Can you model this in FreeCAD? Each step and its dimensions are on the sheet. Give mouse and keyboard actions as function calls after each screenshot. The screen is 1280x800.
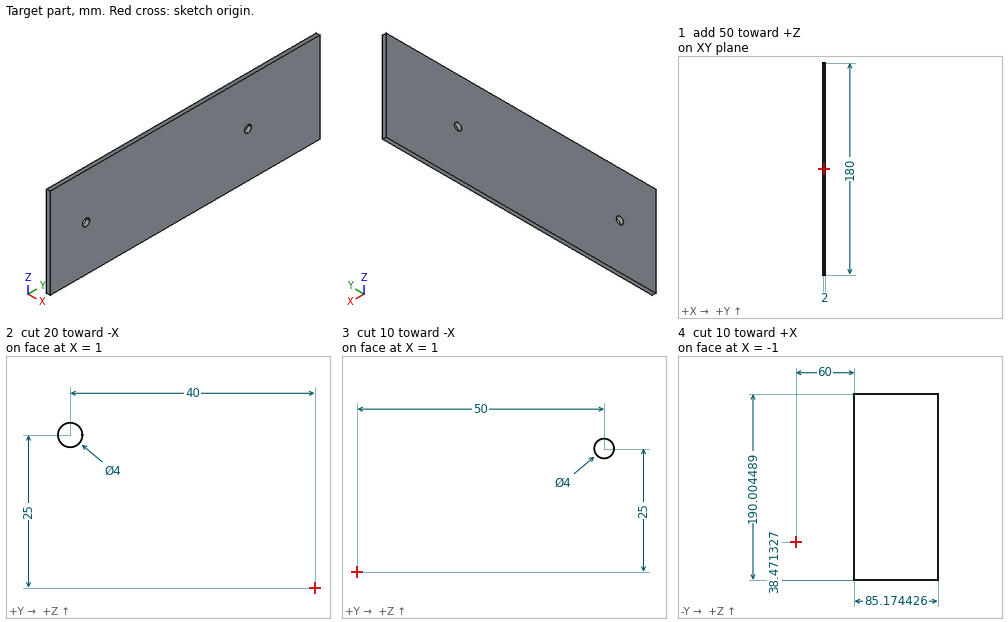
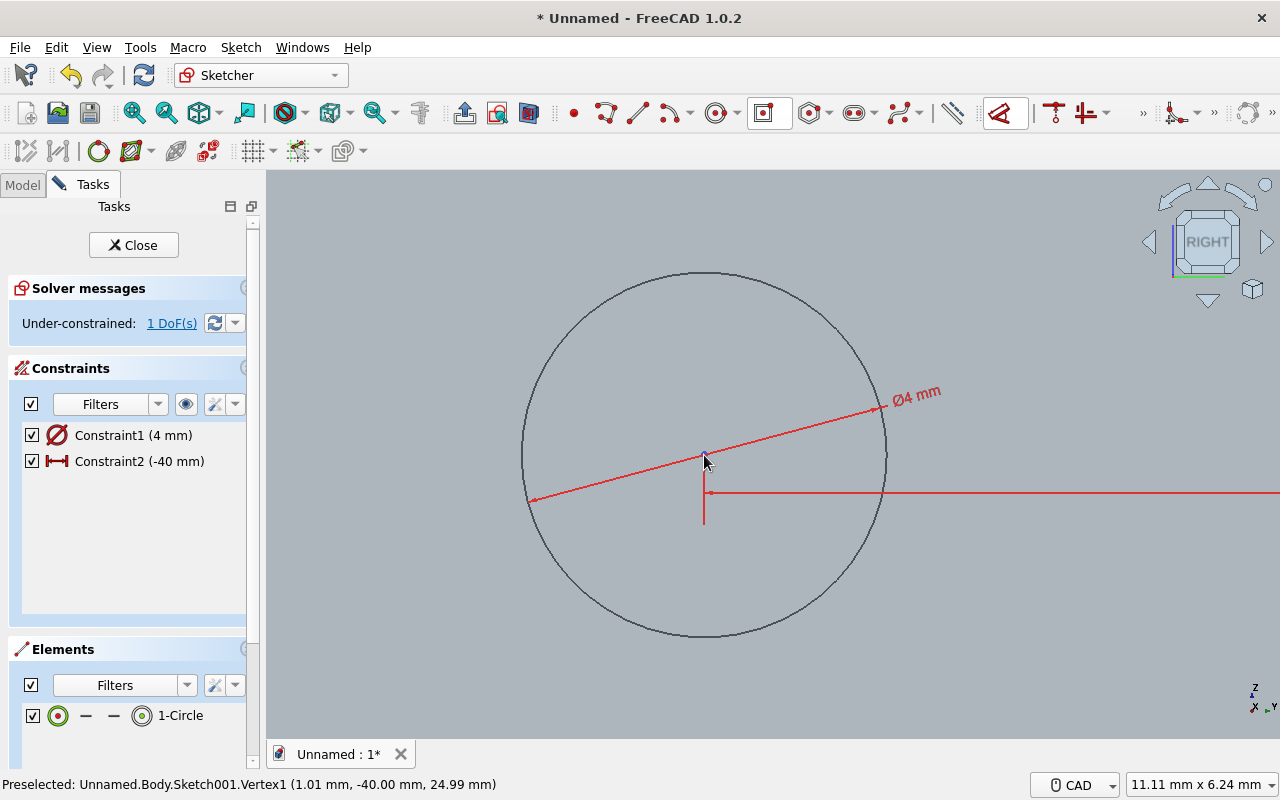
click(704, 455)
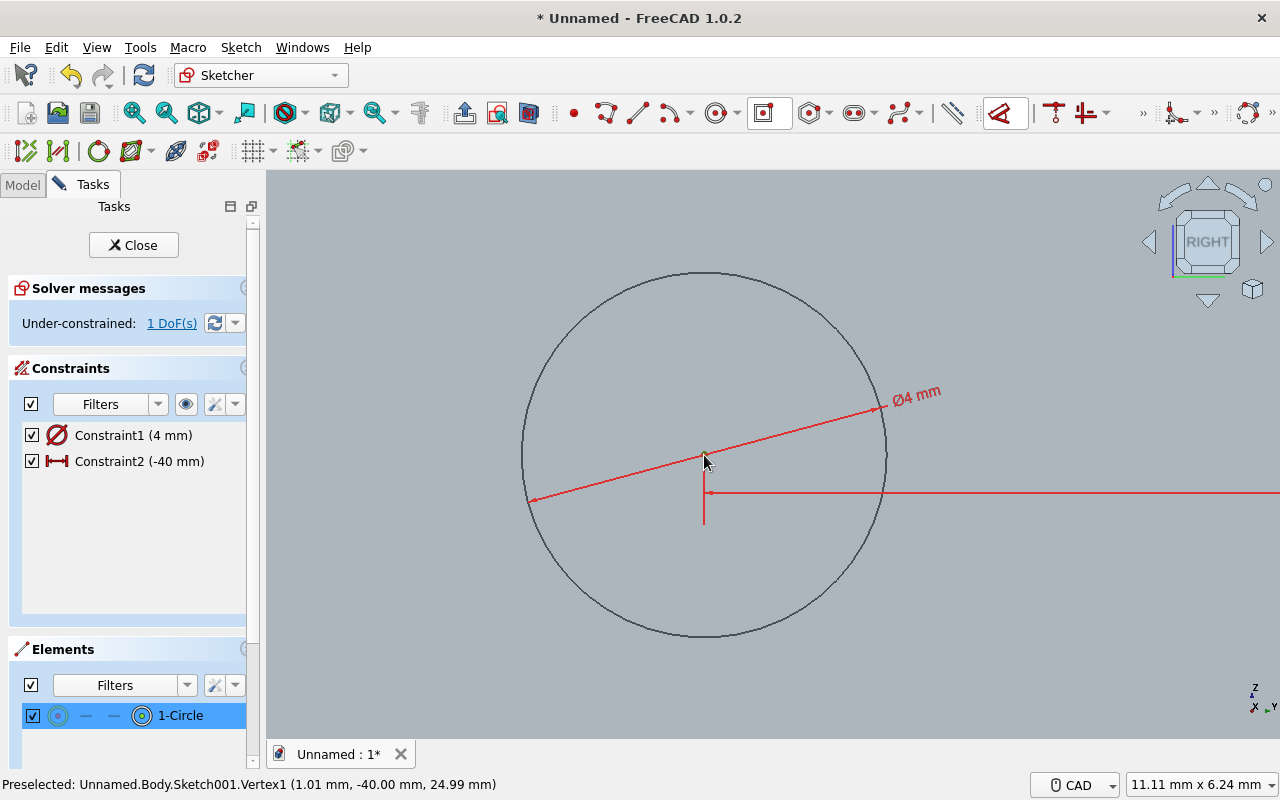
click(1022, 114)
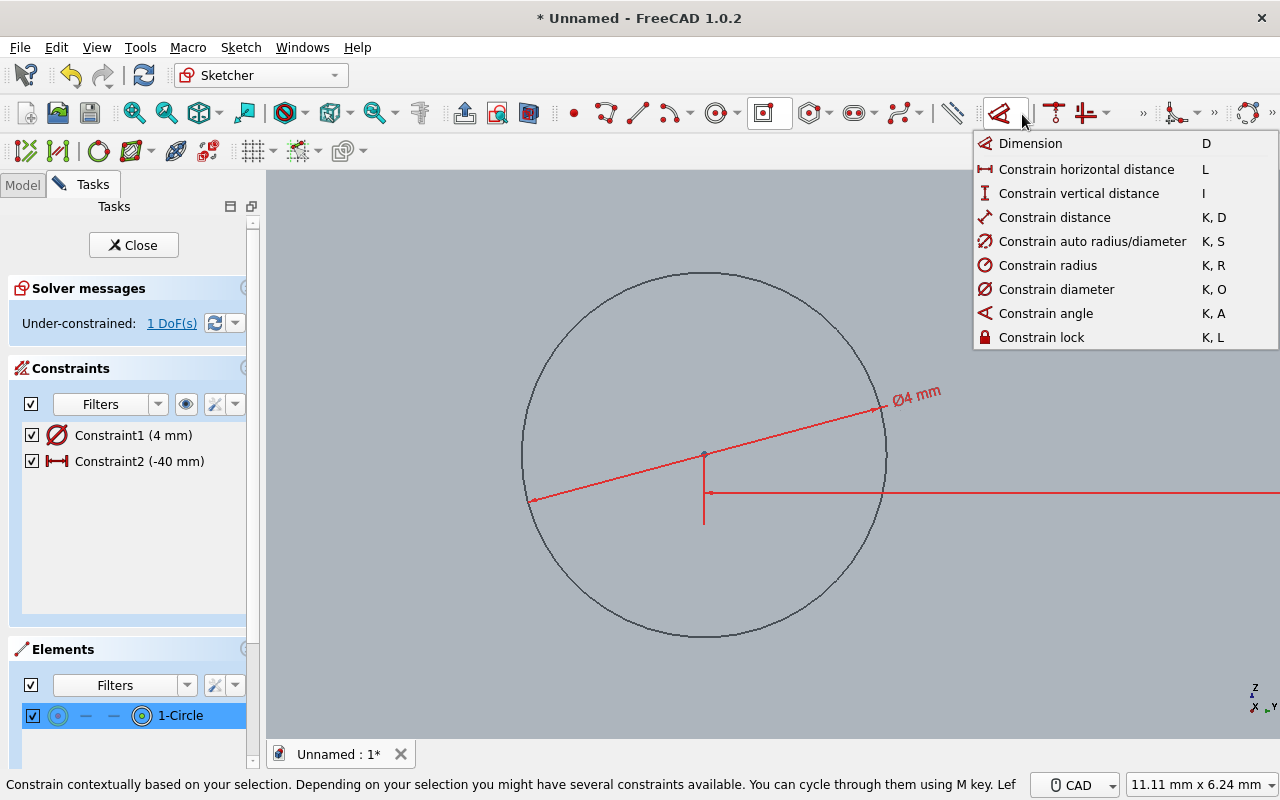
click(1126, 193)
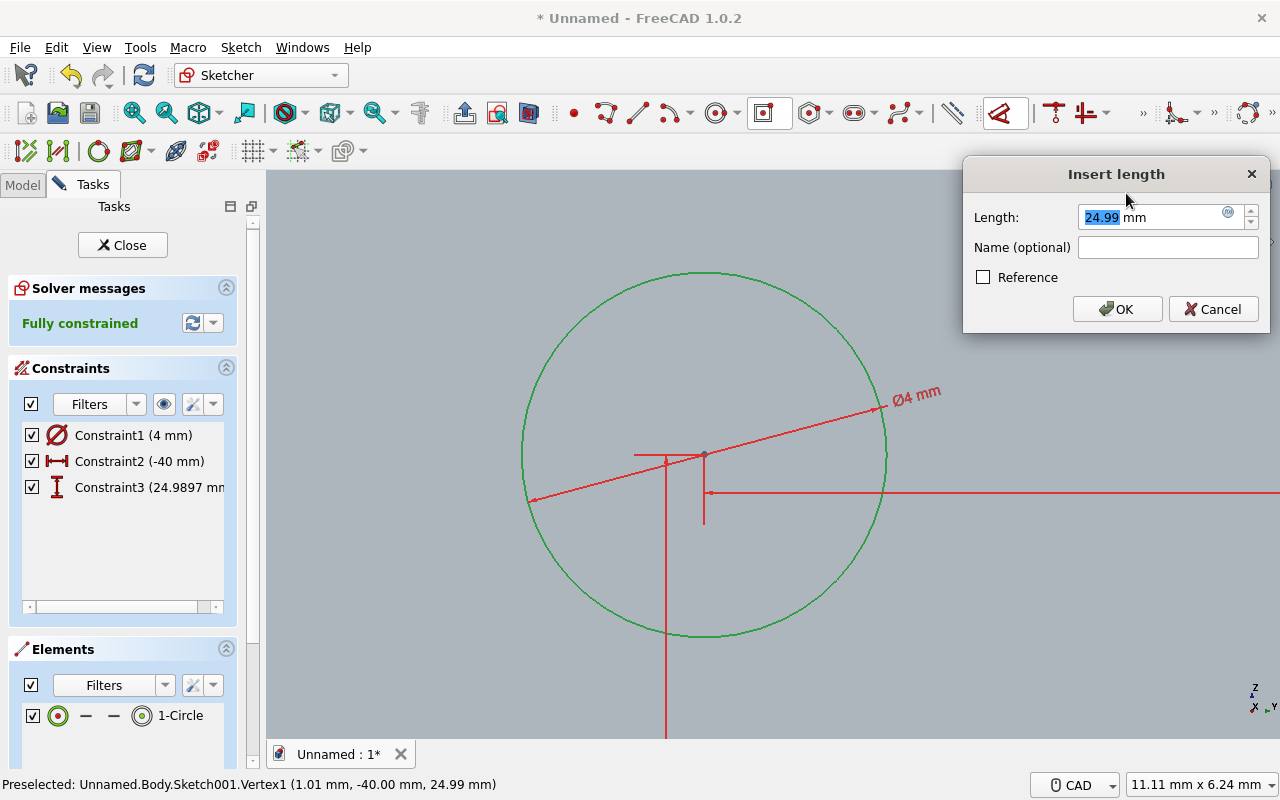
text(25)
key(Return)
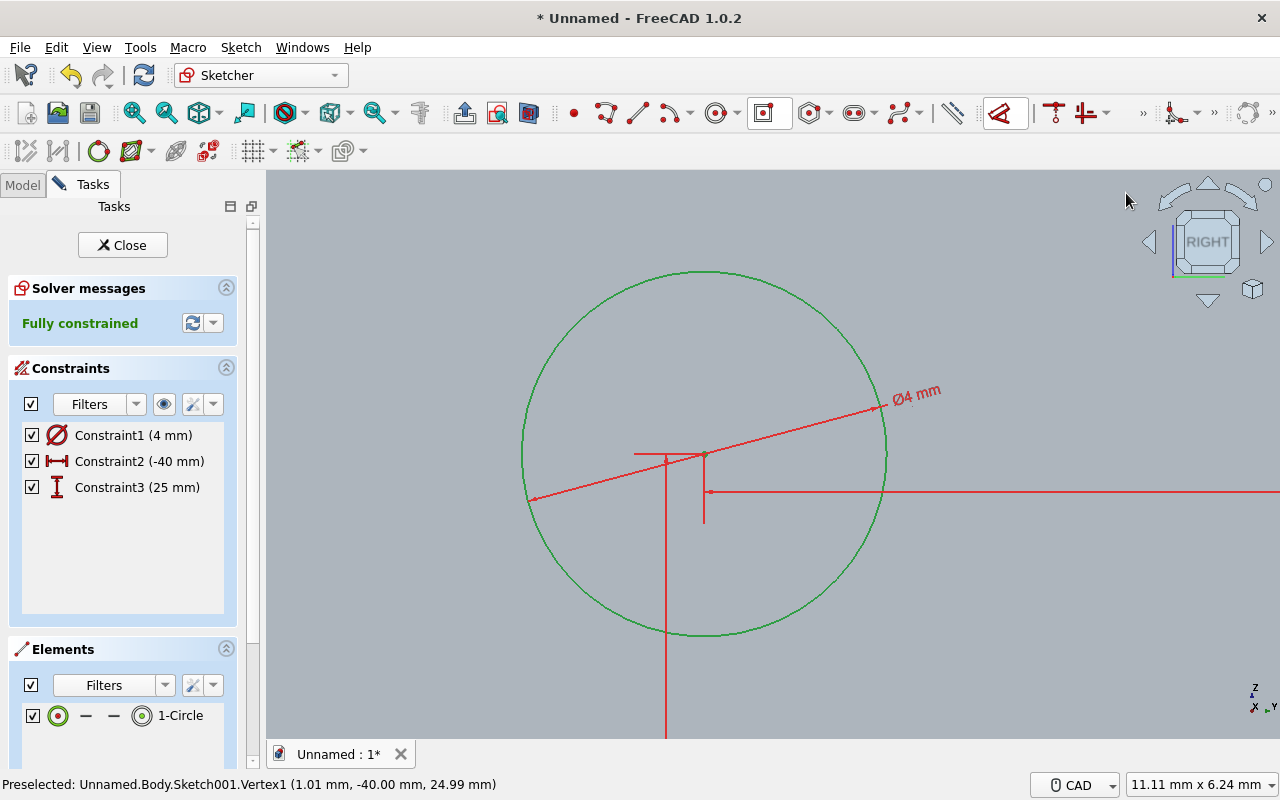
click(123, 245)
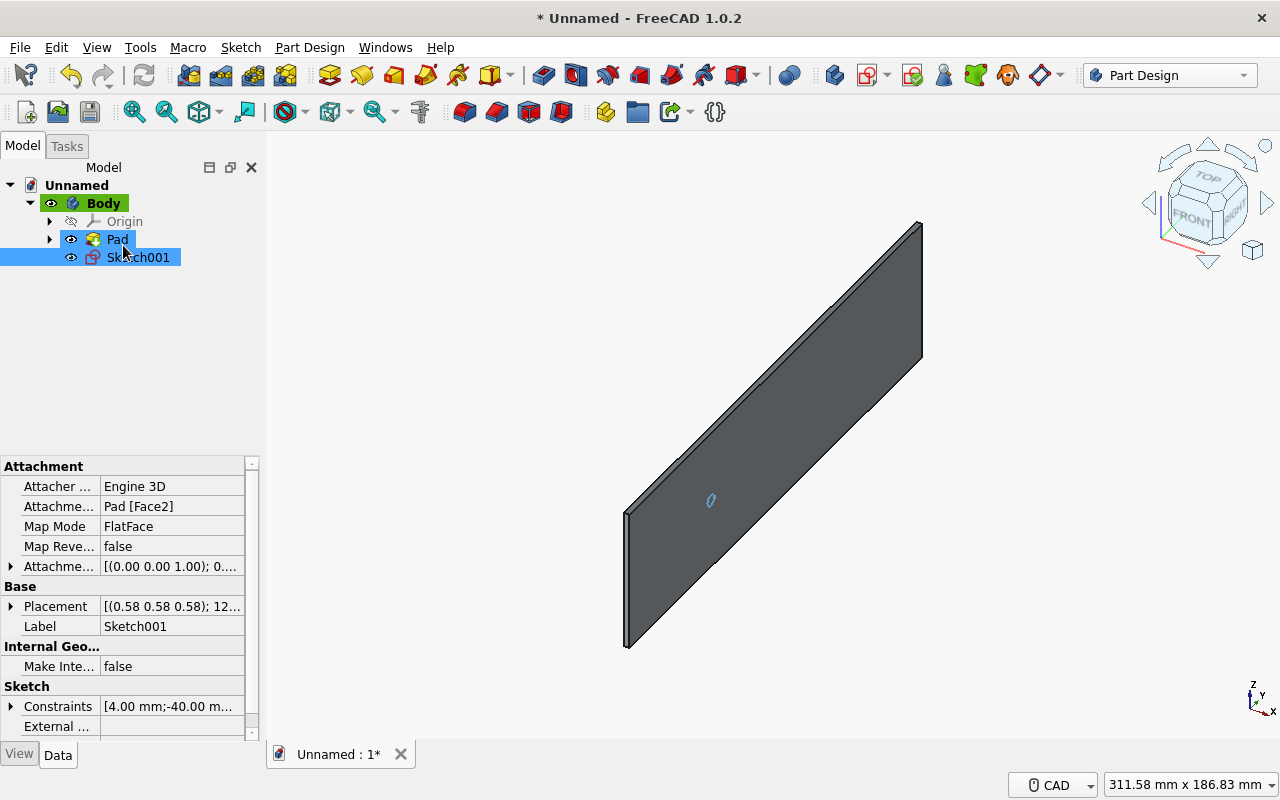
click(544, 76)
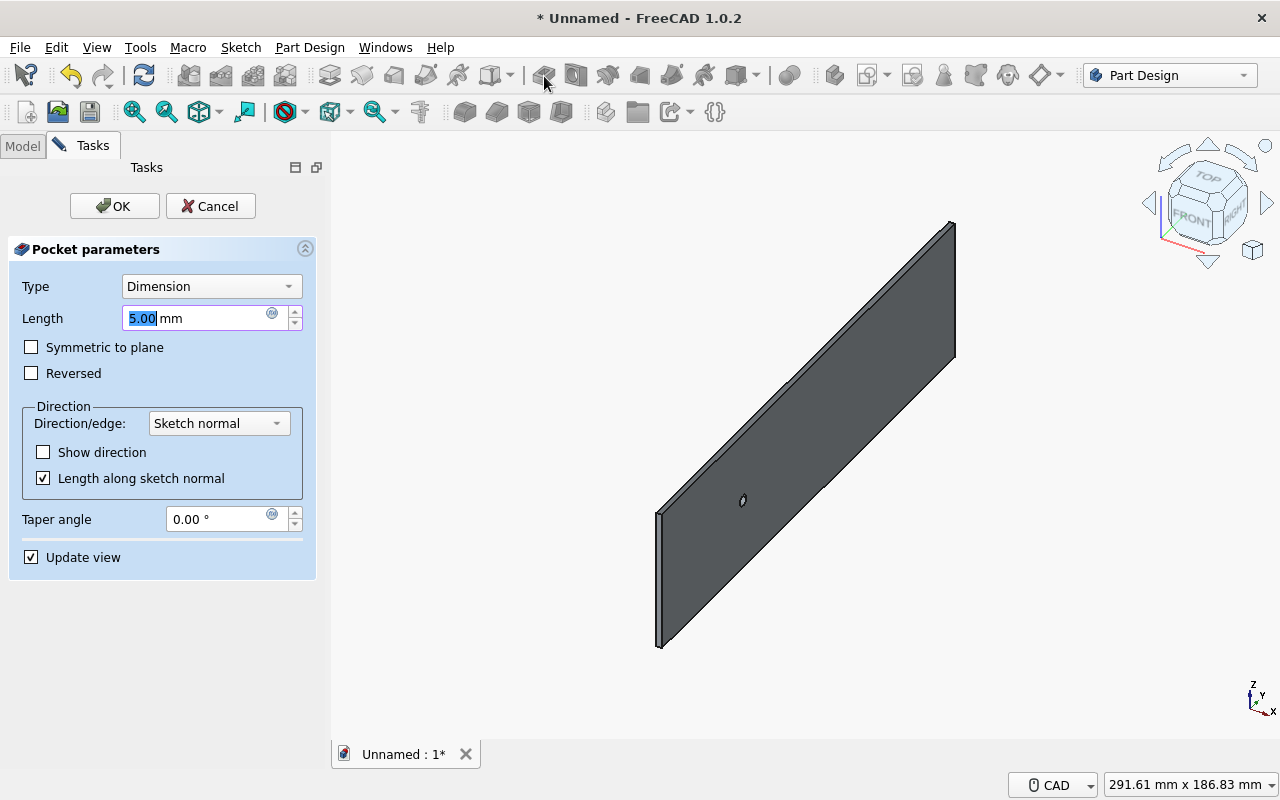
text(20)
key(Tab)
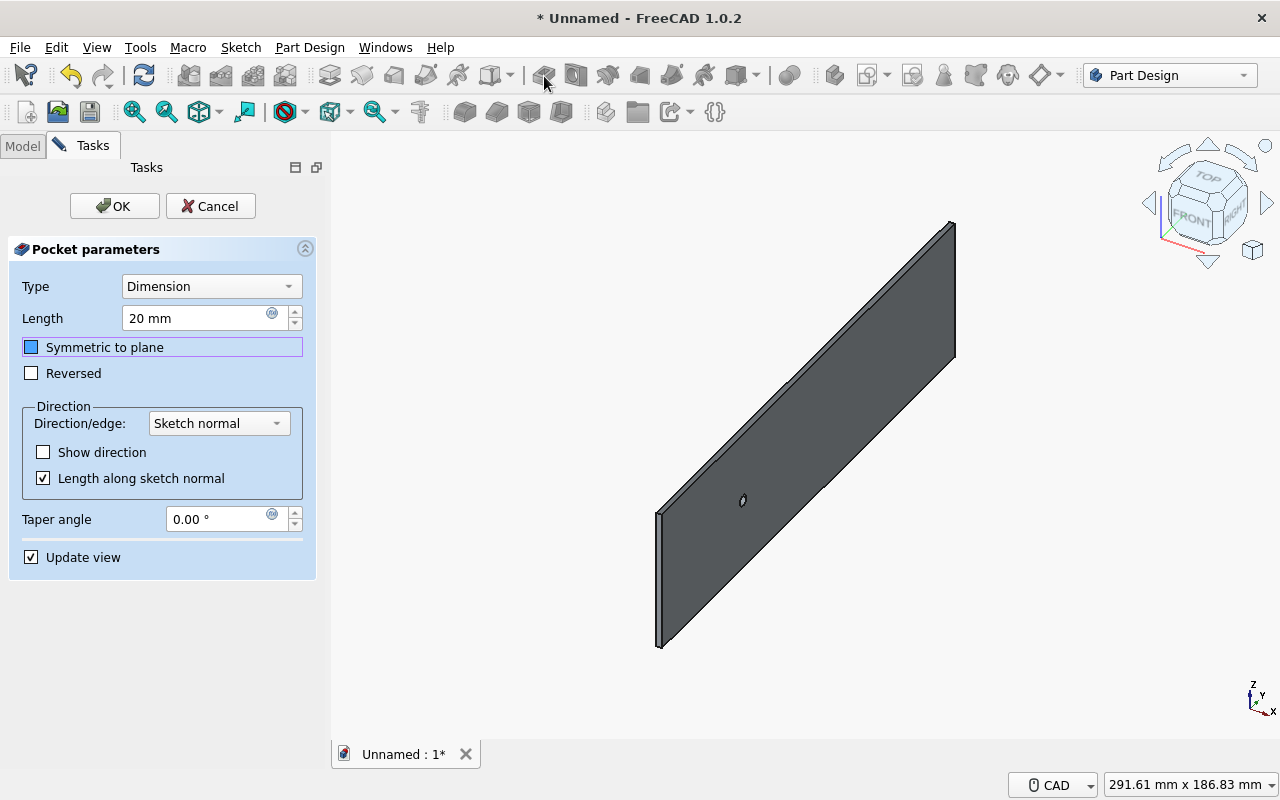
click(115, 206)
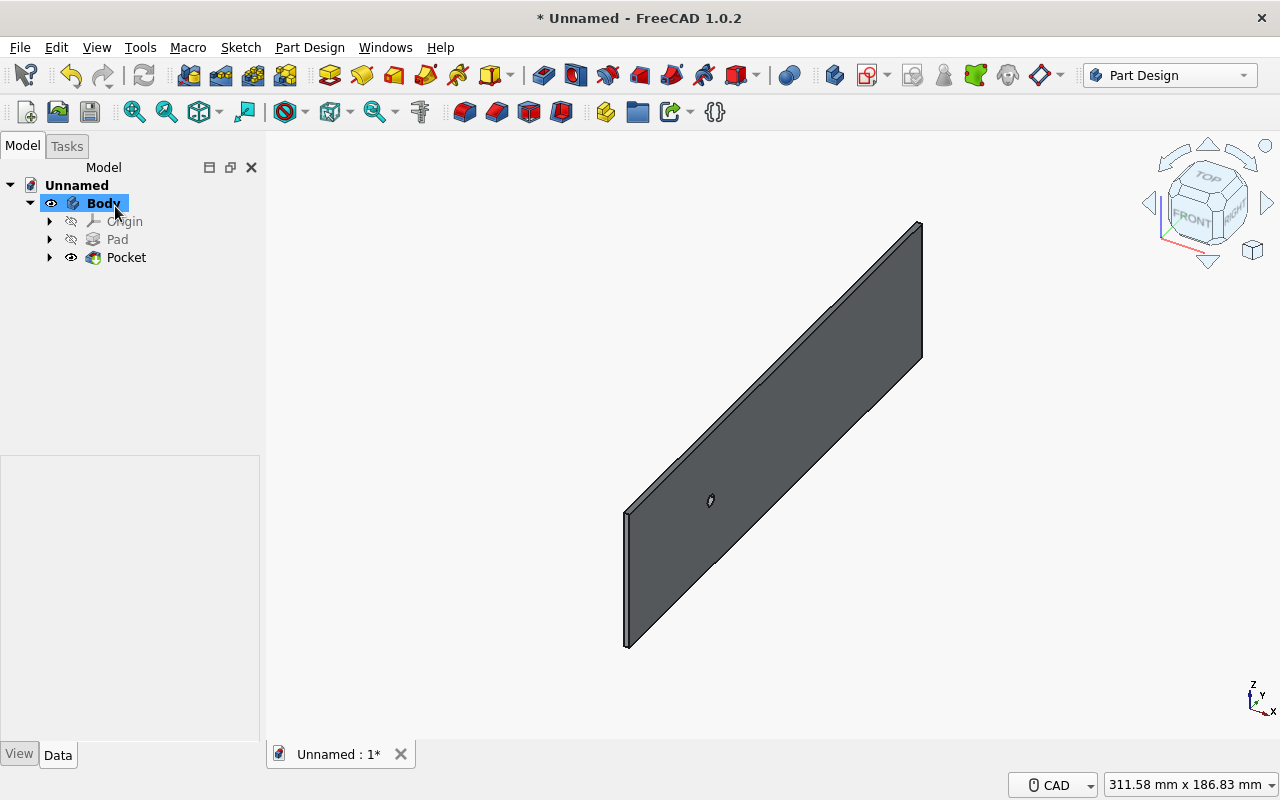
click(860, 352)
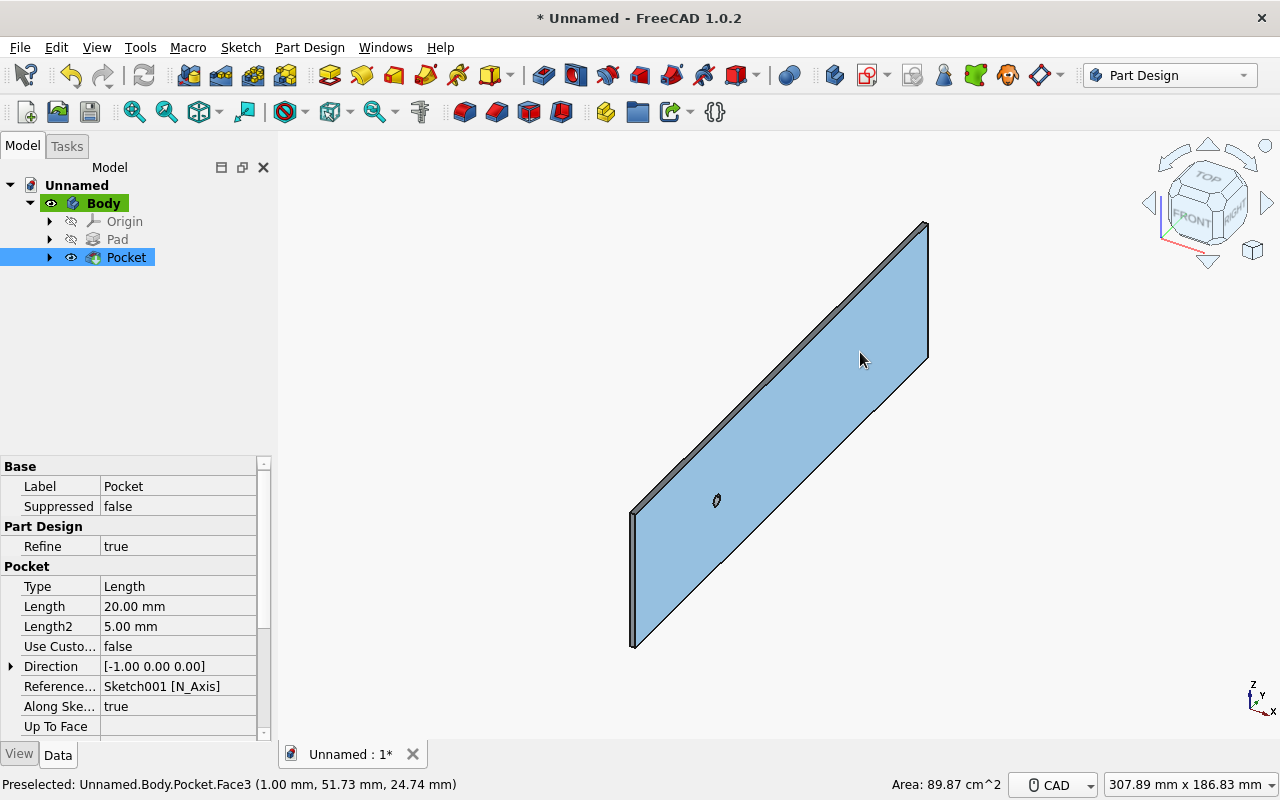
click(868, 76)